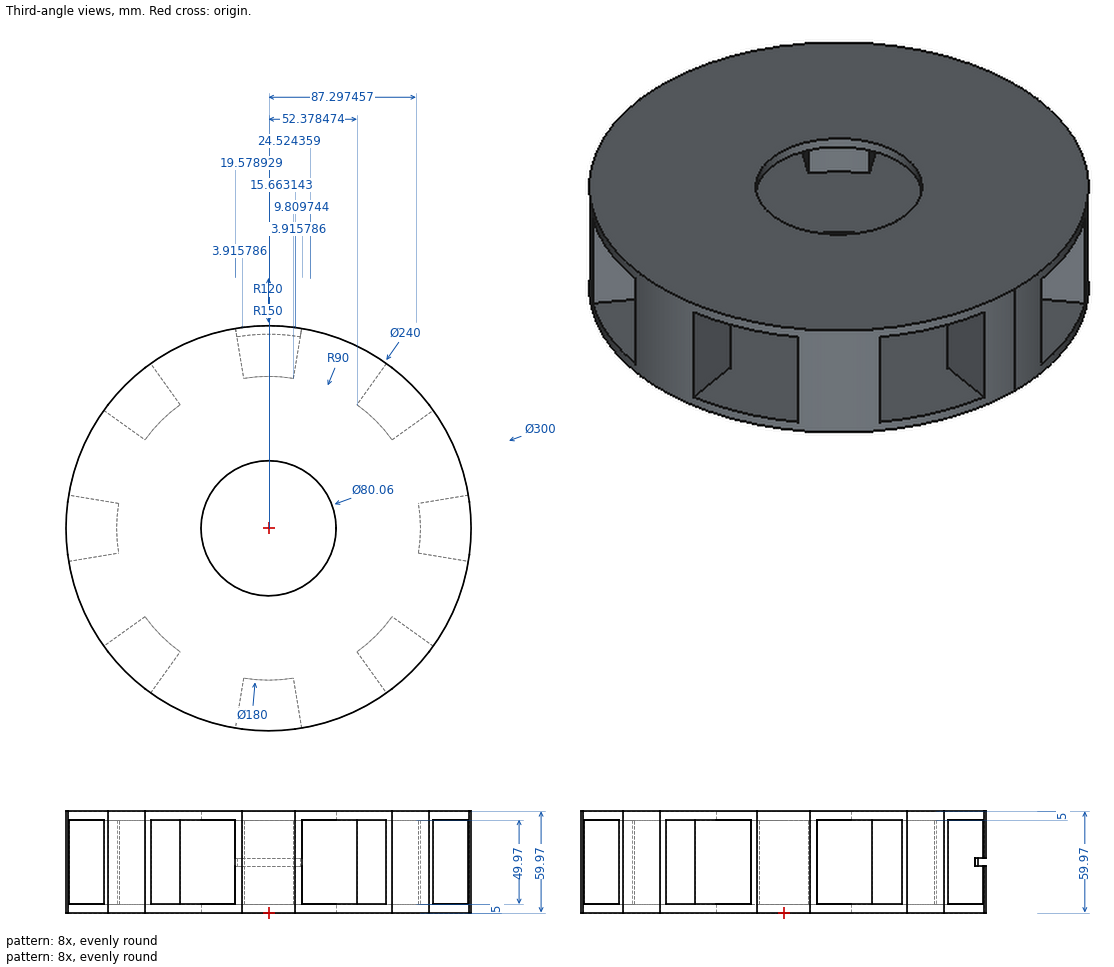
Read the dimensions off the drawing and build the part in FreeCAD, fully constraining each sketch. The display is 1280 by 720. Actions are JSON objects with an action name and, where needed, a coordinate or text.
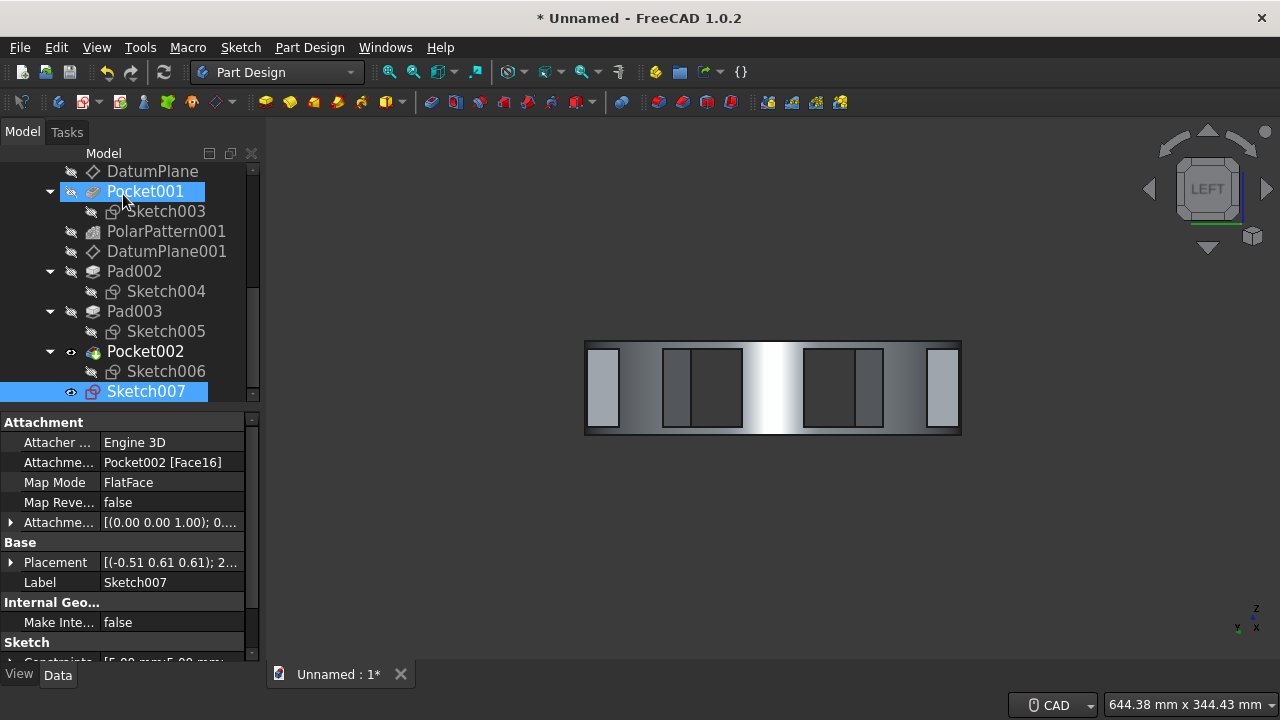
{"action": "left_click", "coordinate": [480, 102]}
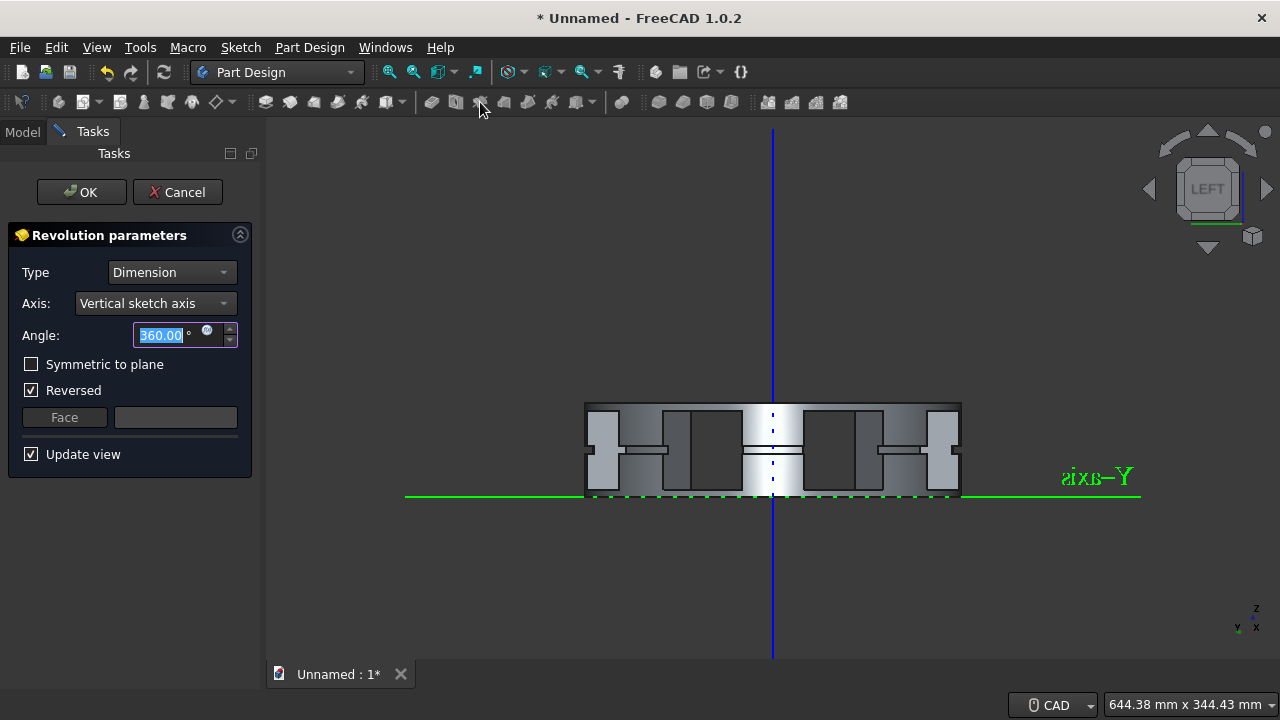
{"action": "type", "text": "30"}
{"action": "key", "text": "Tab"}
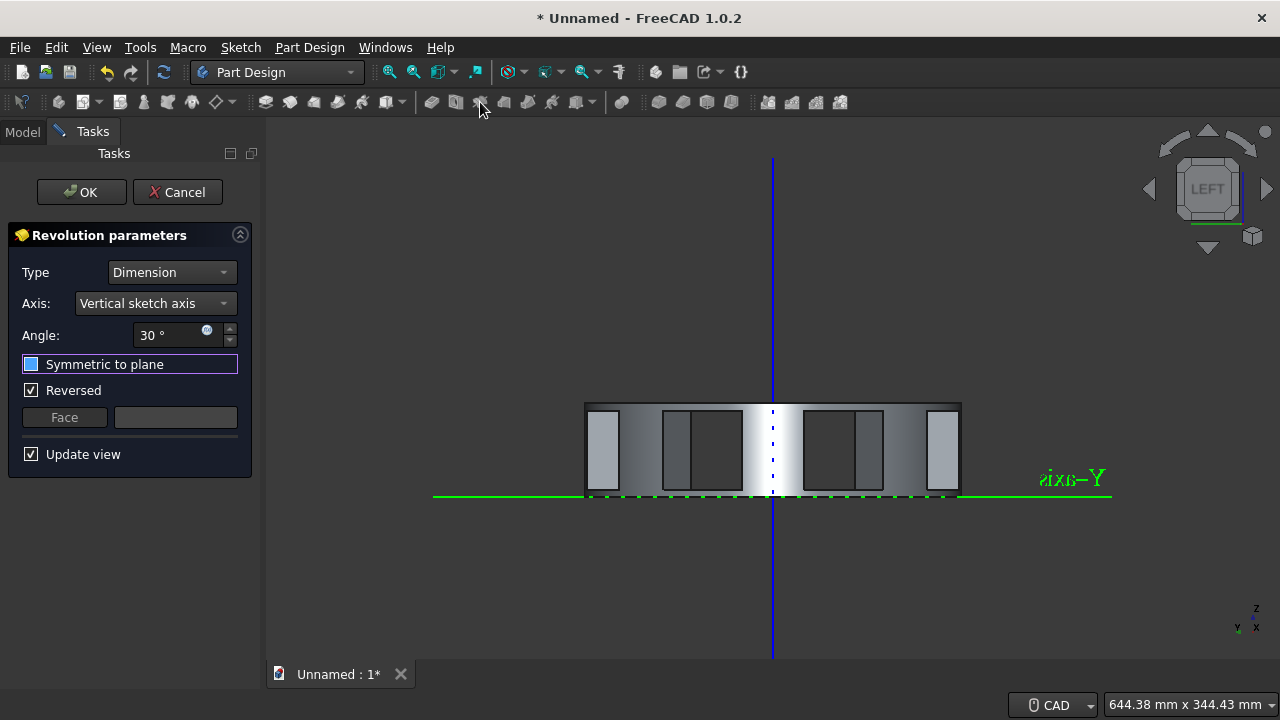
{"action": "left_click", "coordinate": [30, 390]}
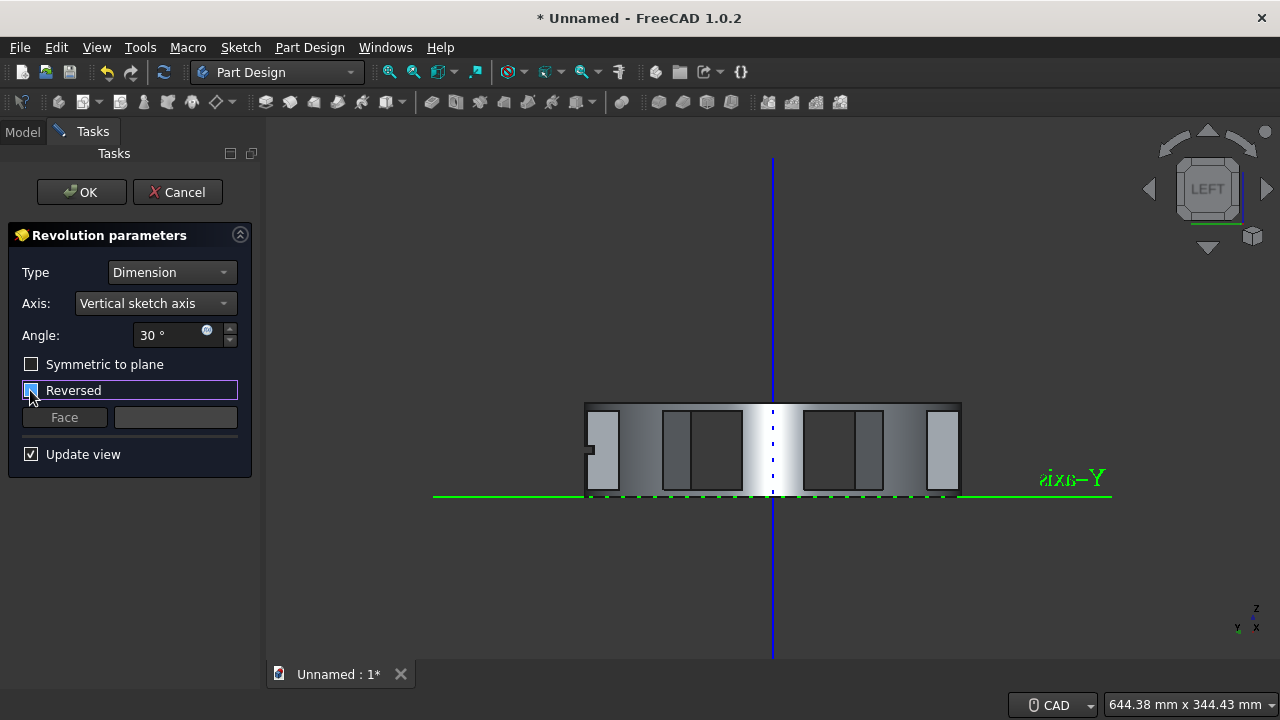
{"action": "left_click", "coordinate": [82, 192]}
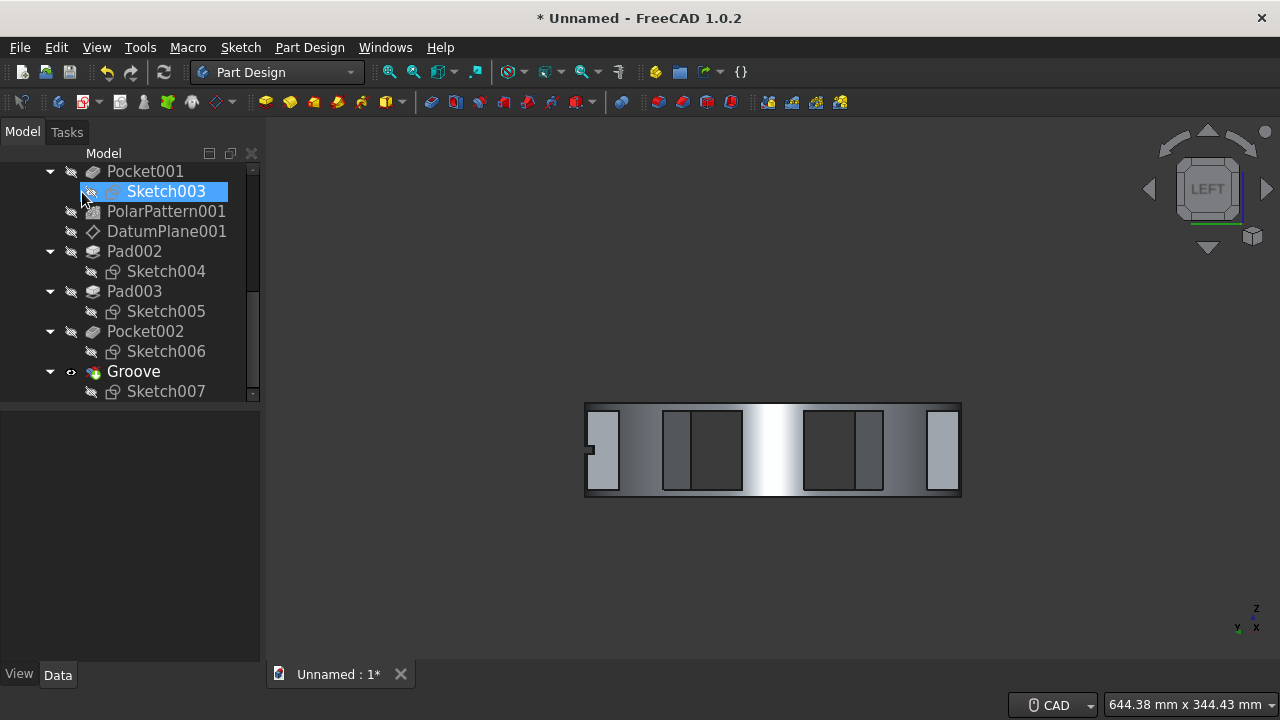
{"action": "key", "text": "0"}